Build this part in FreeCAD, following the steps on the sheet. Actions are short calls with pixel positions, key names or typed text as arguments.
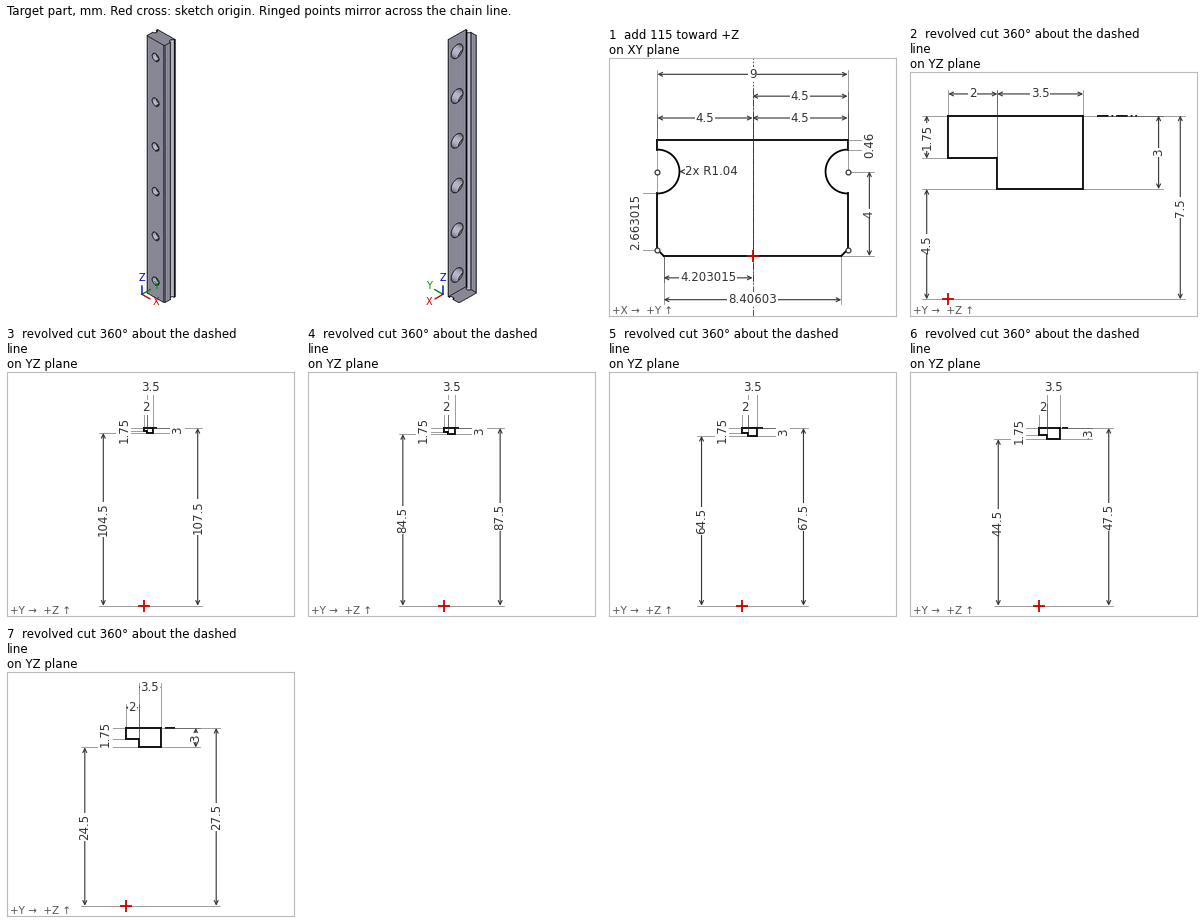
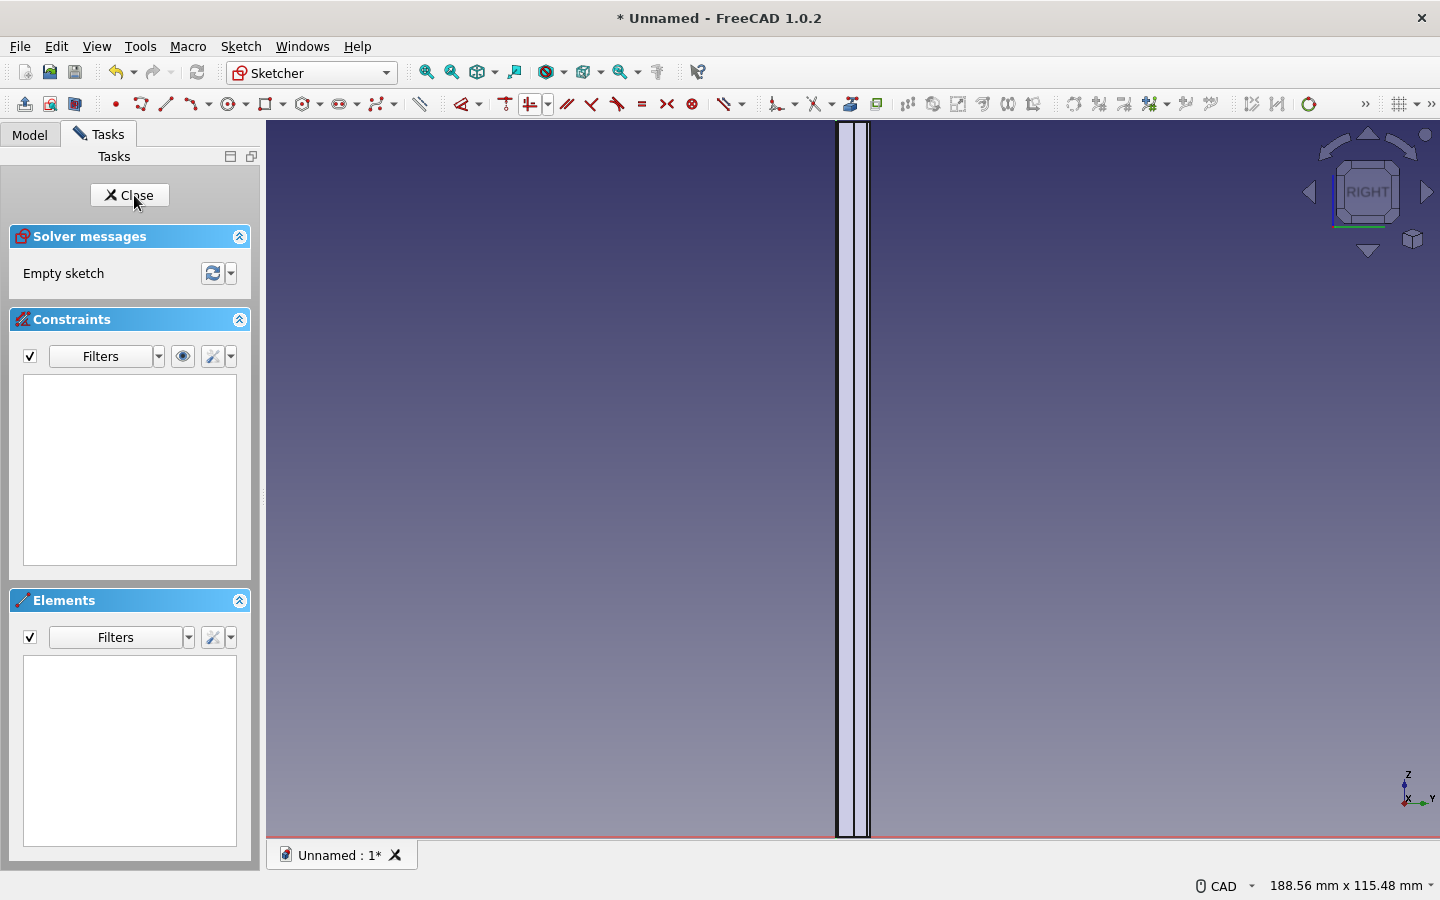
key(q)
key(s)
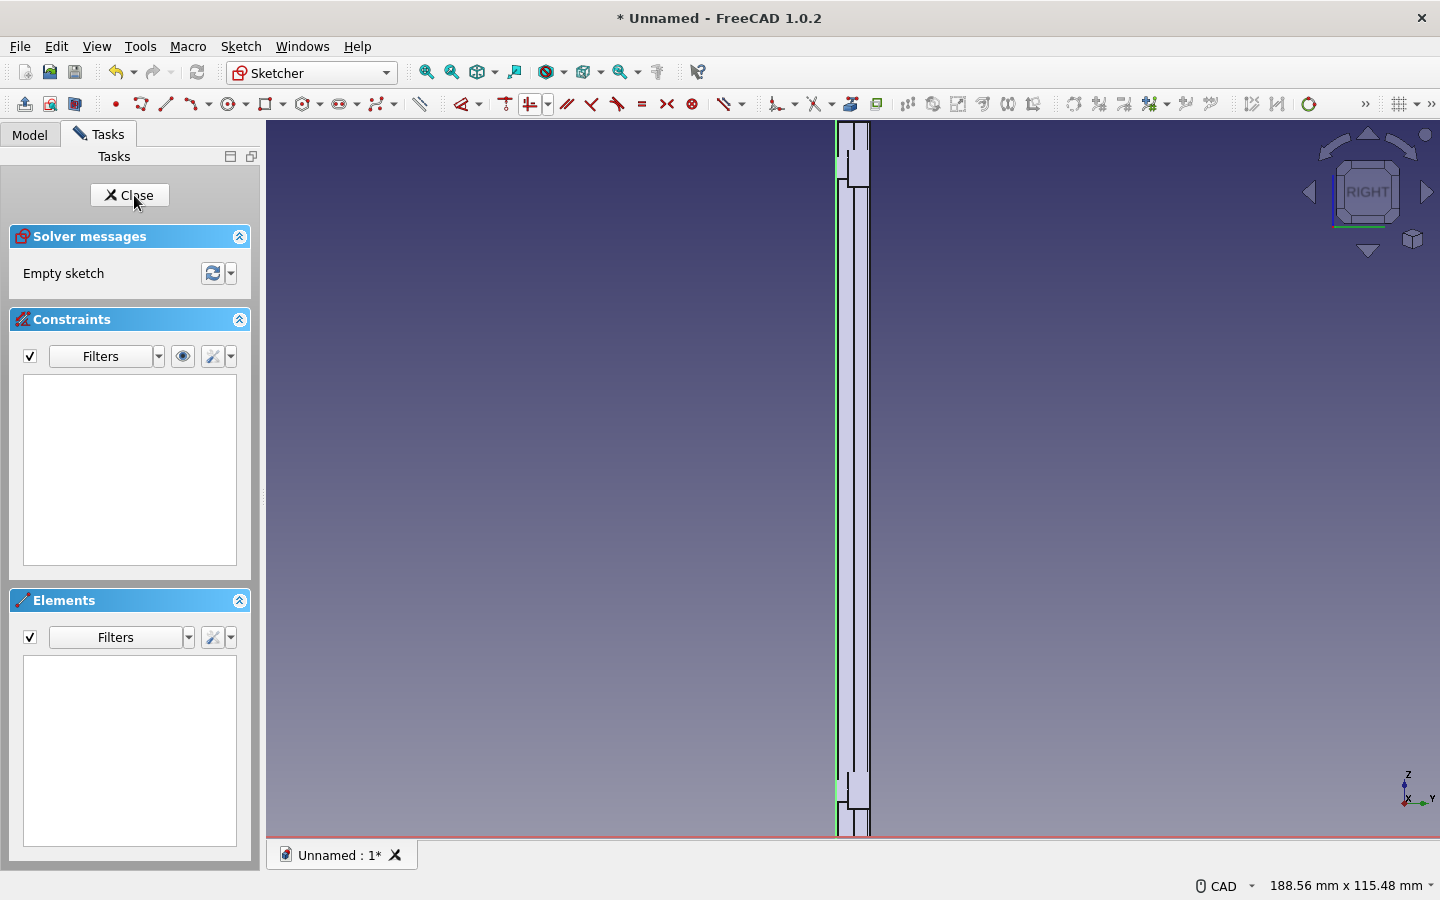
scroll(866, 288, up, 13)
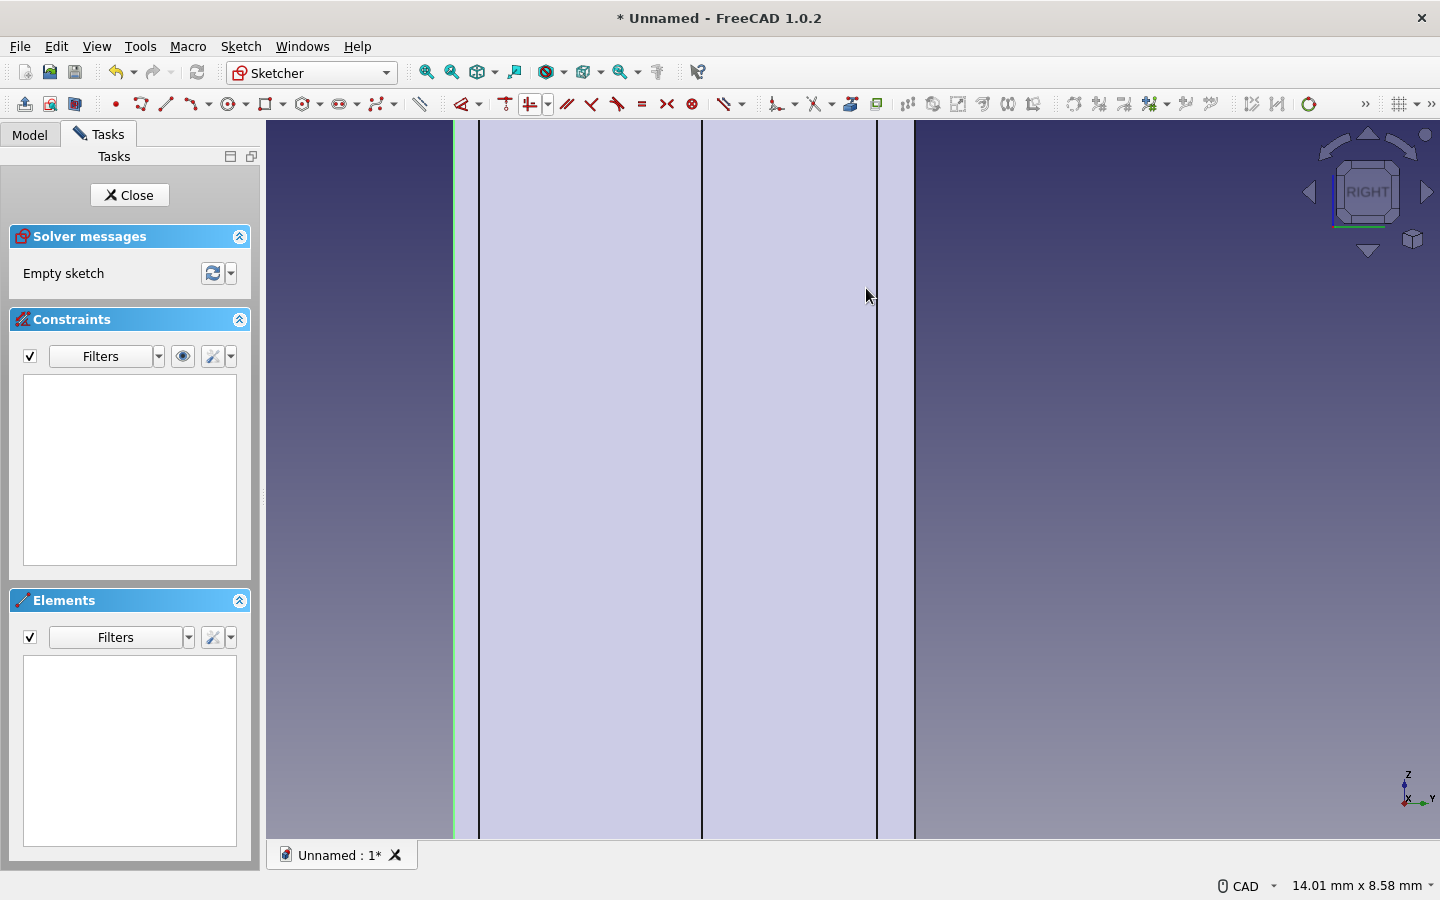
click(141, 104)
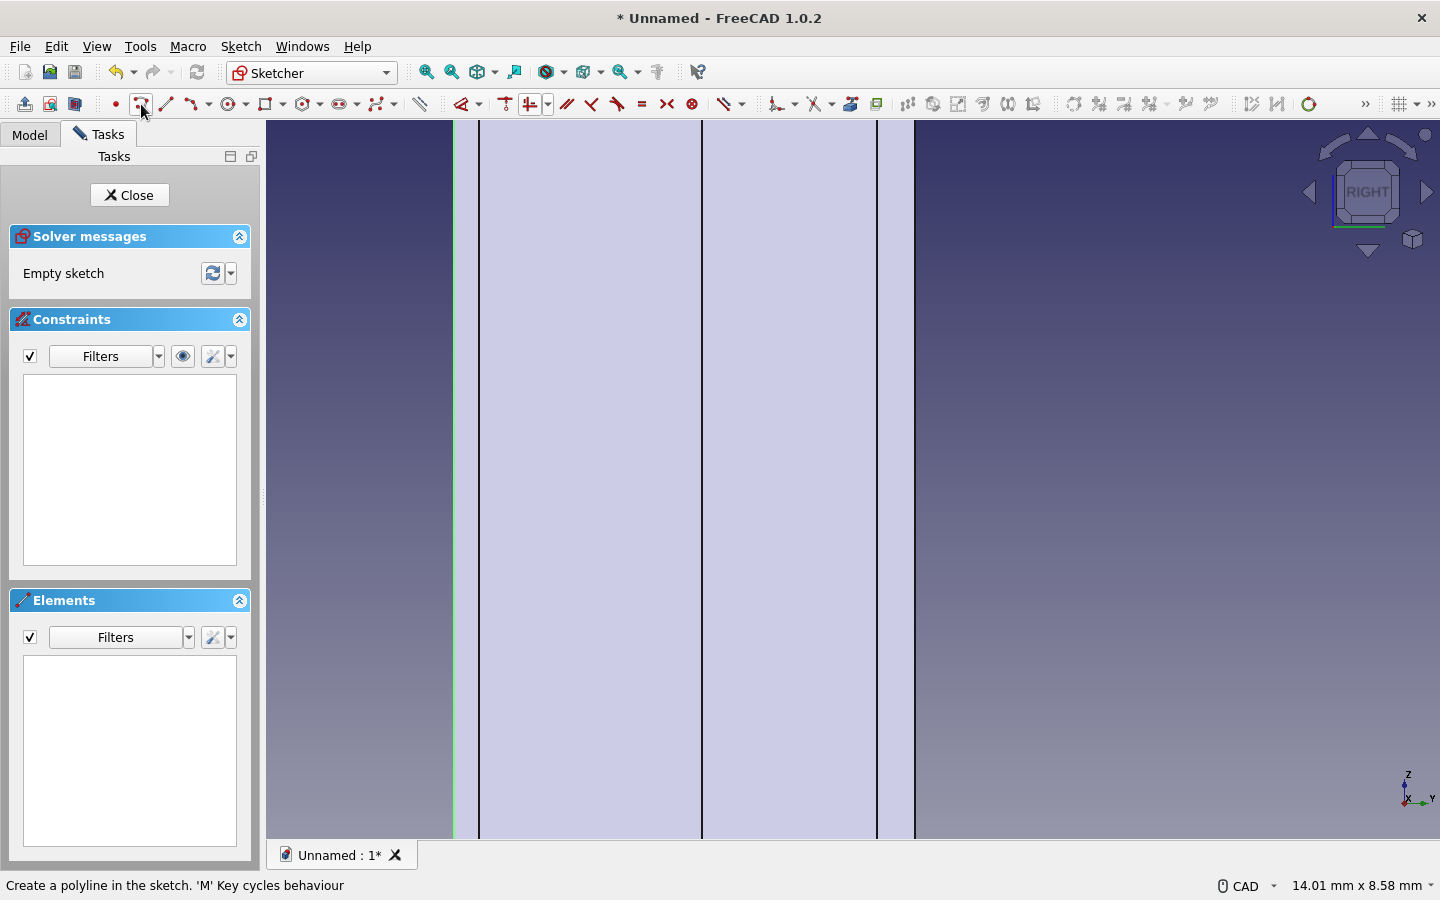
click(622, 600)
click(915, 600)
click(915, 349)
click(454, 349)
click(463, 495)
click(622, 495)
click(622, 601)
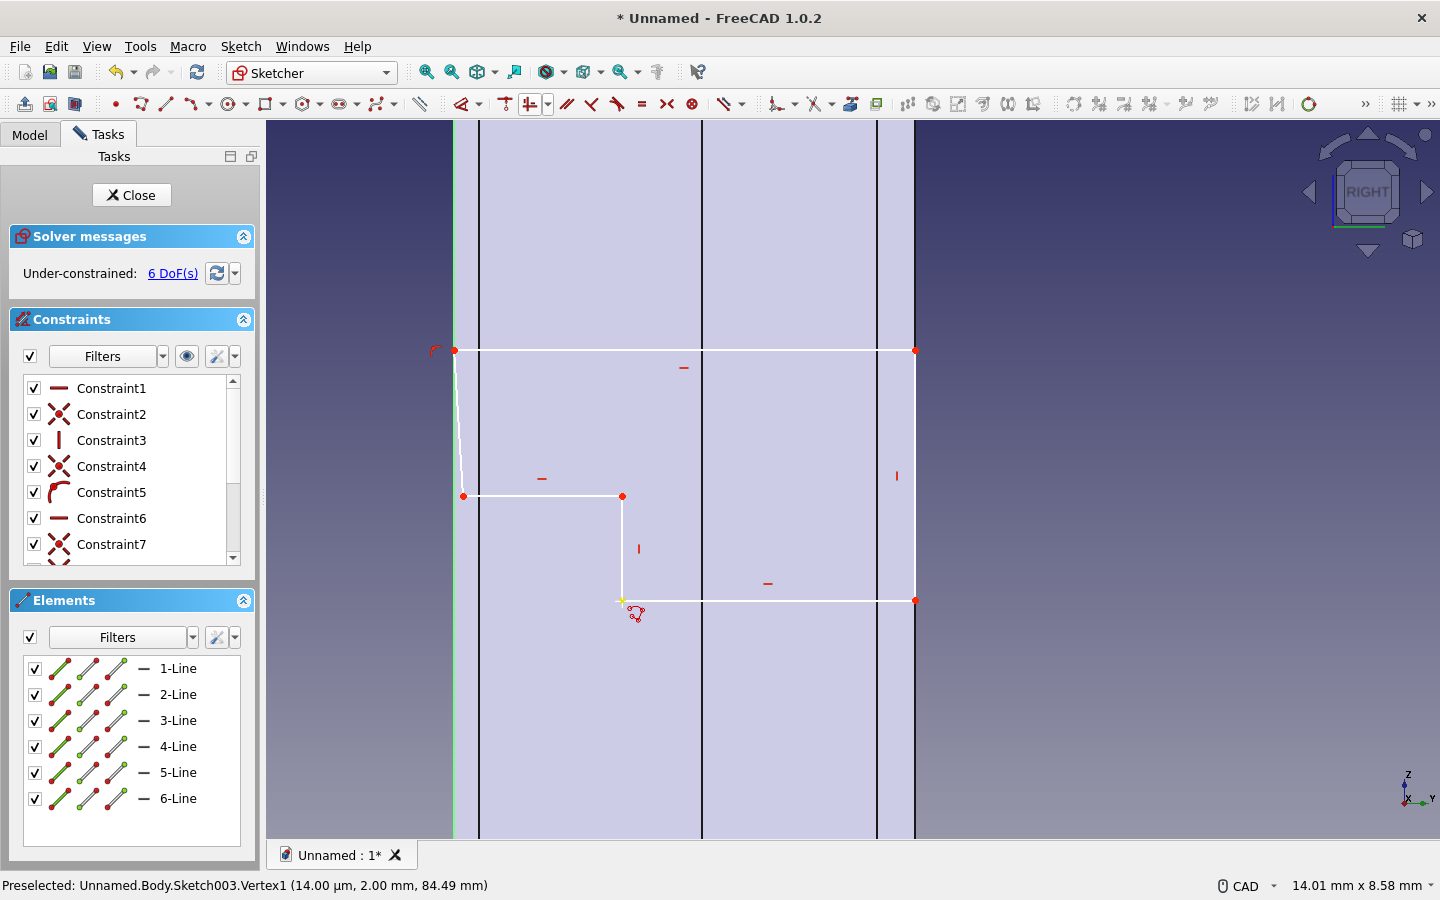
key(g)
key(l)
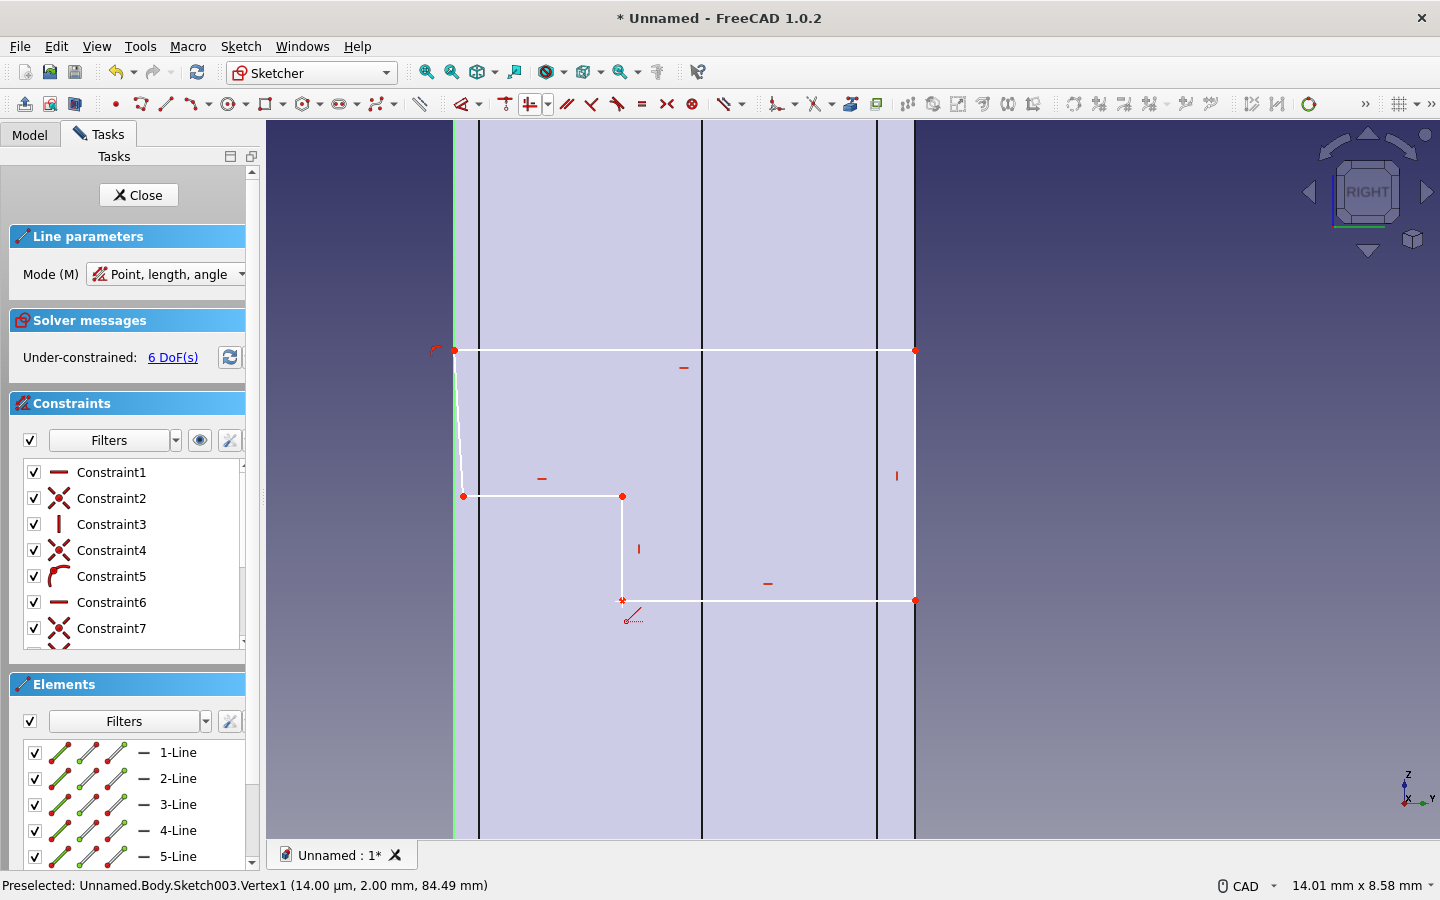
click(961, 349)
click(1100, 349)
key(Escape)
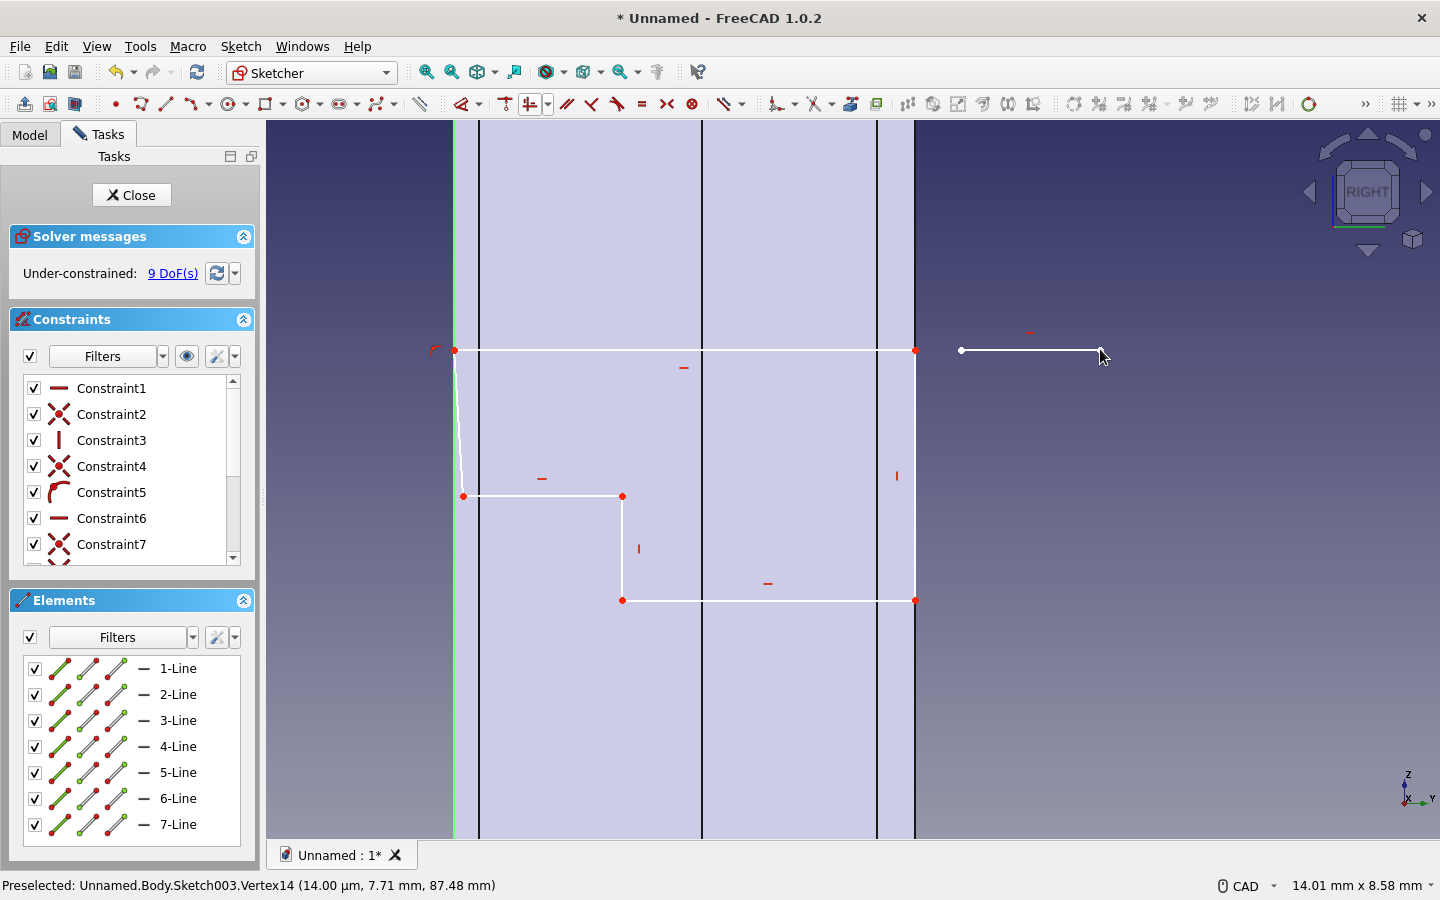
click(1003, 350)